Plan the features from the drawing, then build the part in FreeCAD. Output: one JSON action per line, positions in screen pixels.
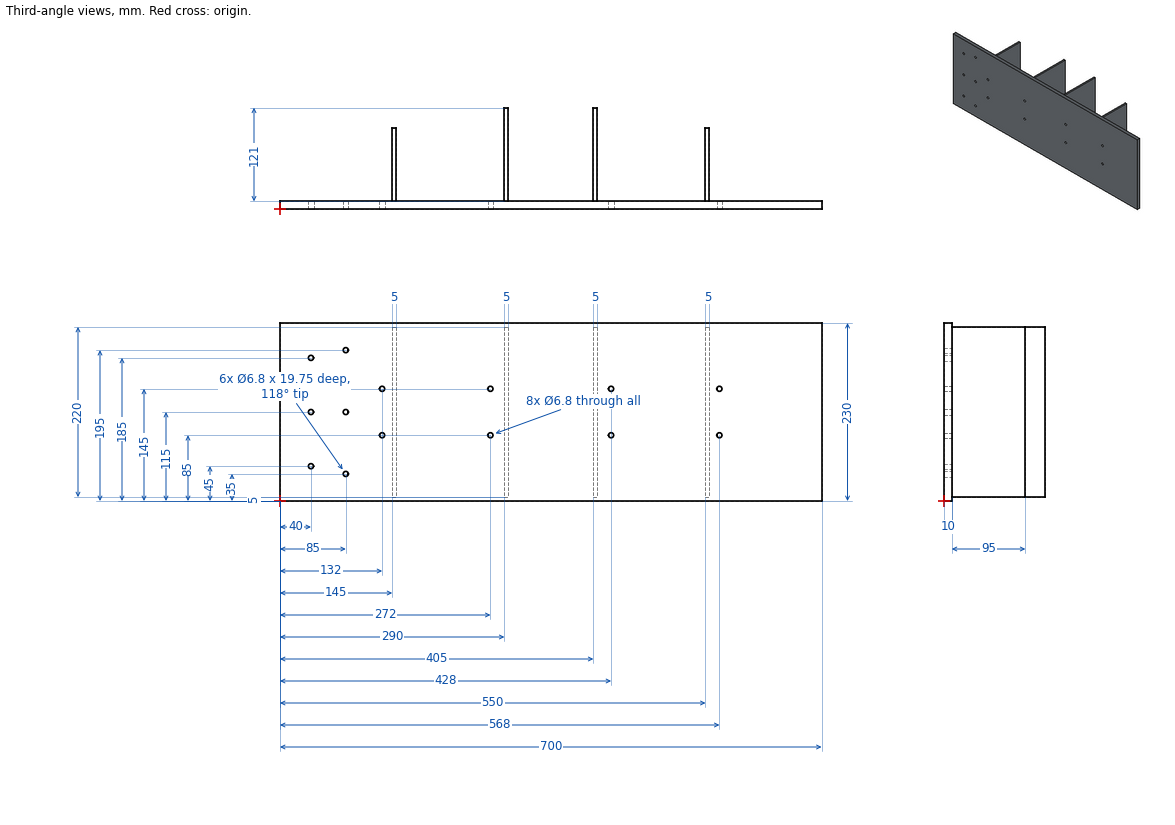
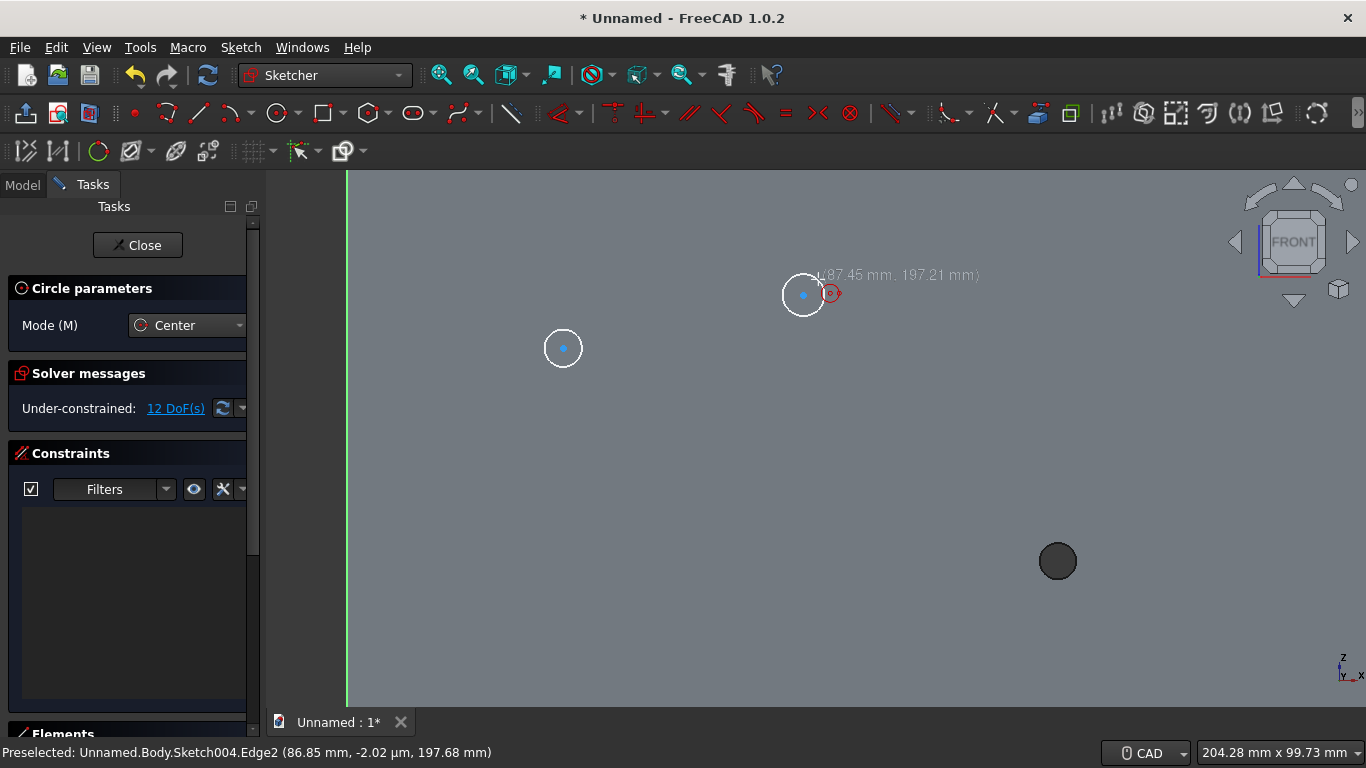
{"action": "scroll", "coordinate": [817, 279], "scroll_direction": "down", "scroll_amount": 6}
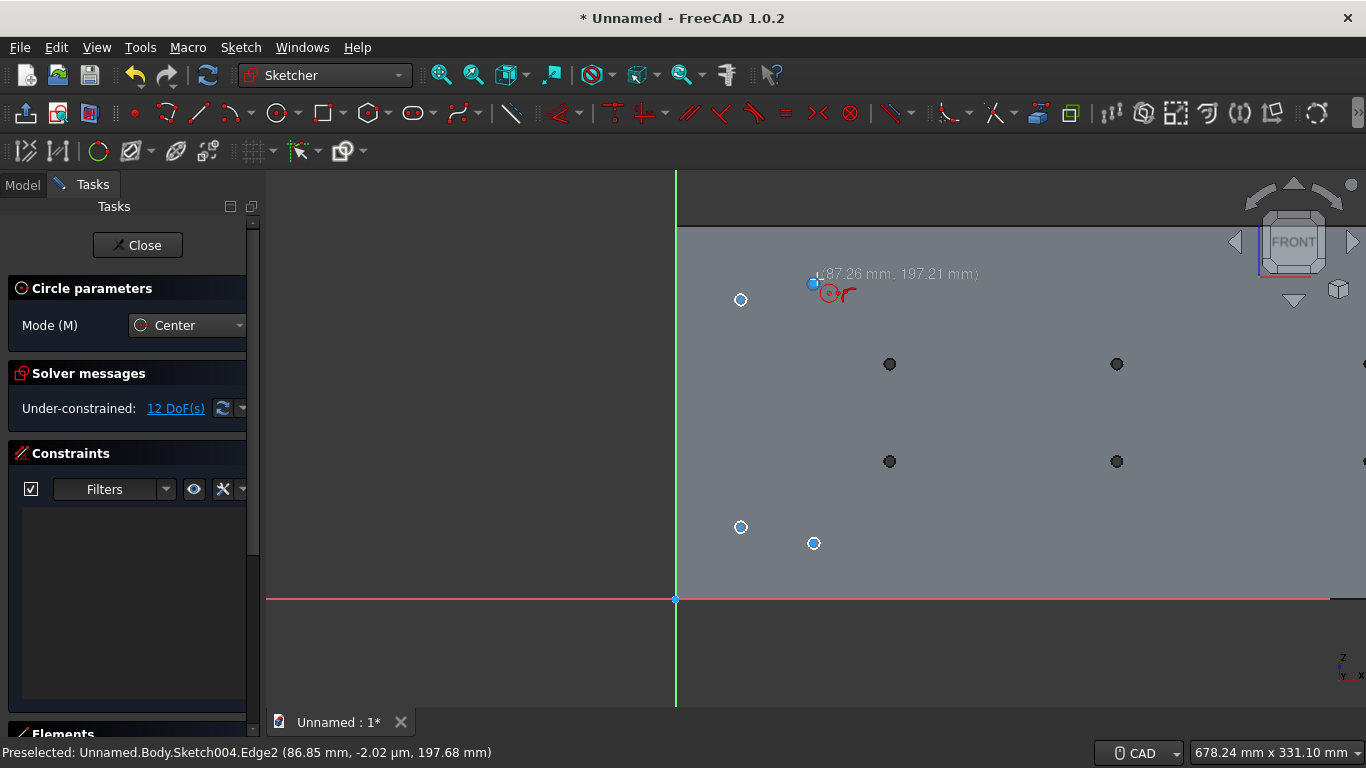
{"action": "scroll", "coordinate": [741, 413], "scroll_direction": "up", "scroll_amount": 8}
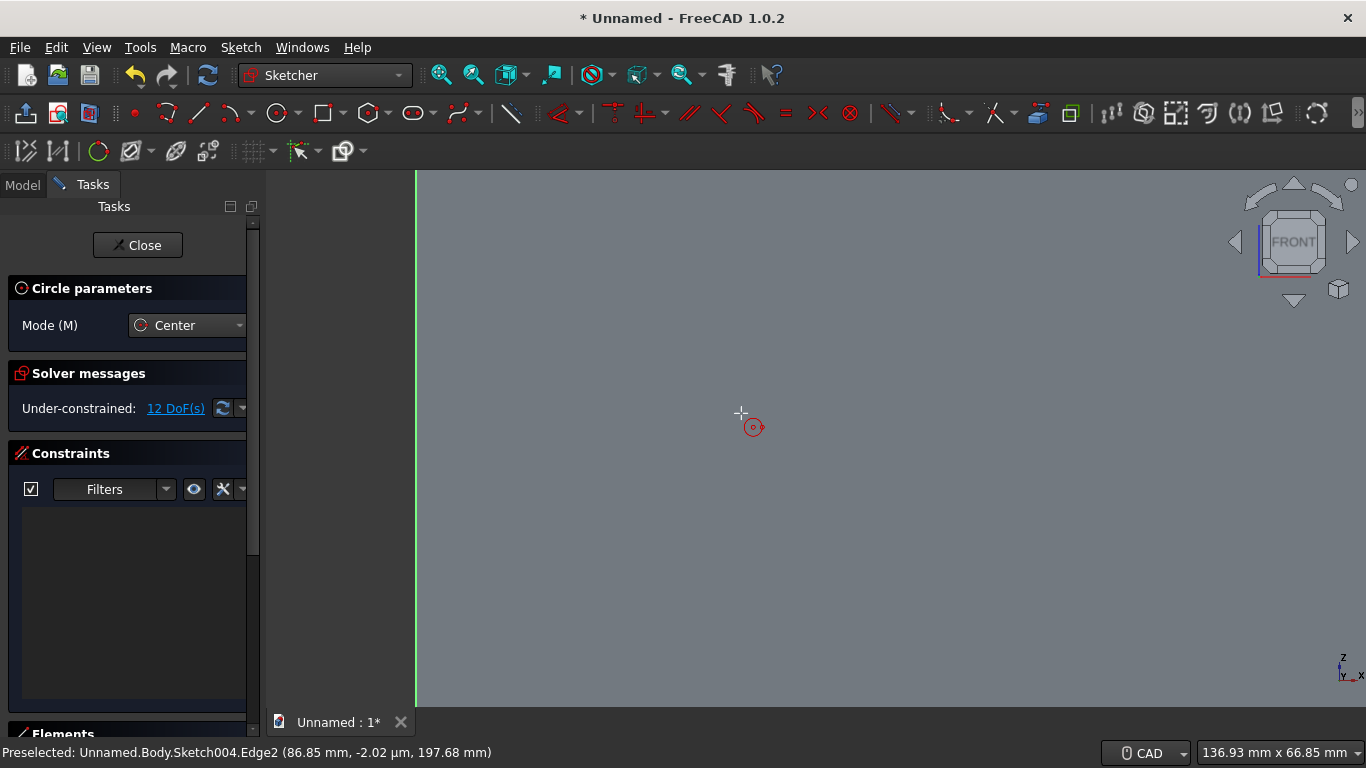
{"action": "scroll", "coordinate": [741, 414], "scroll_direction": "down", "scroll_amount": 8}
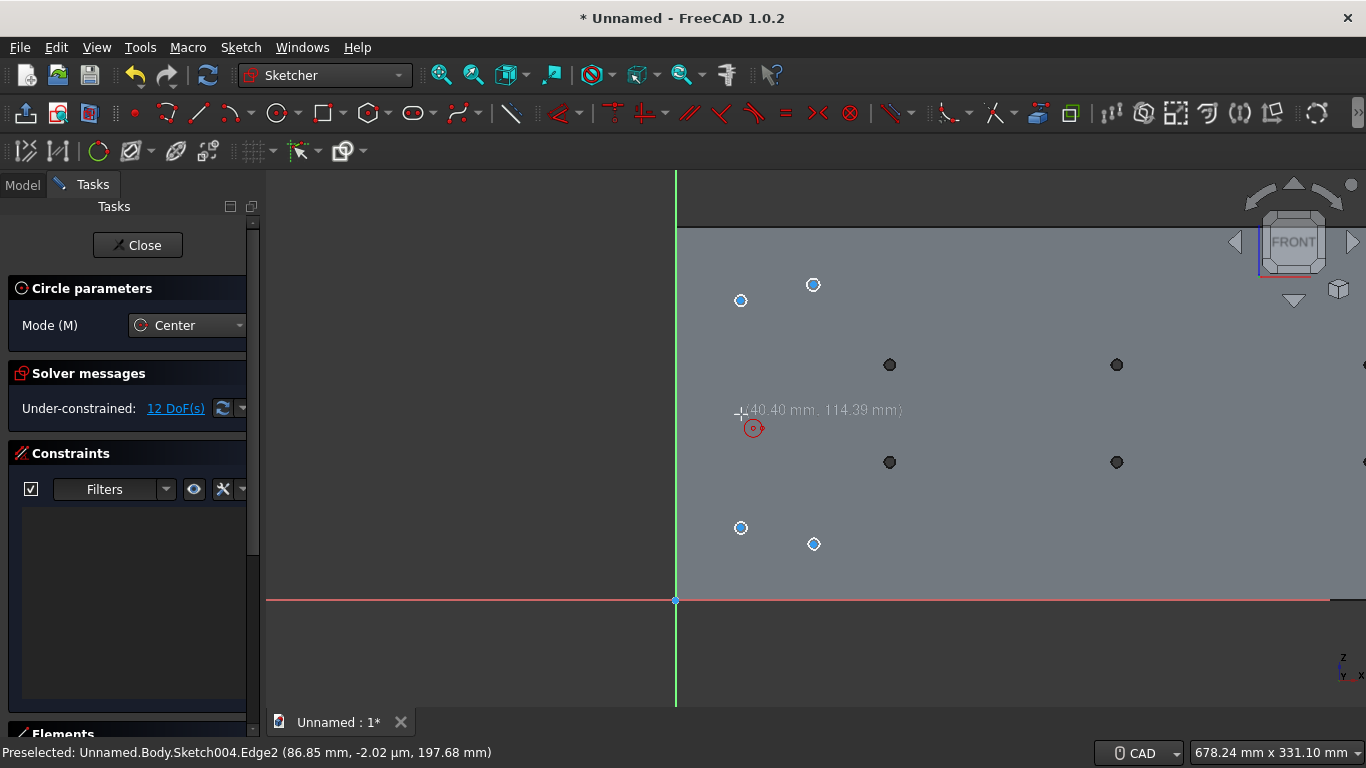
{"action": "left_click", "coordinate": [741, 414]}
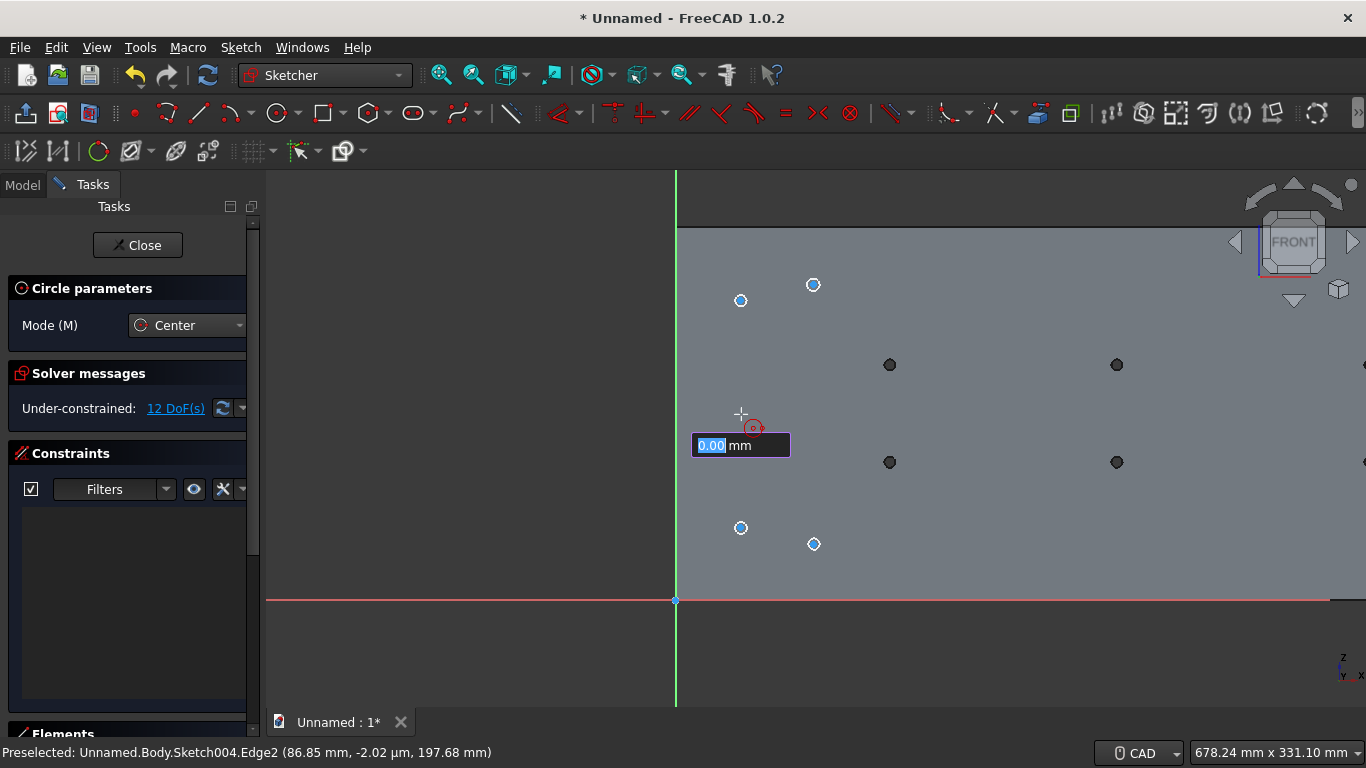
{"action": "scroll", "coordinate": [745, 410], "scroll_direction": "up", "scroll_amount": 6}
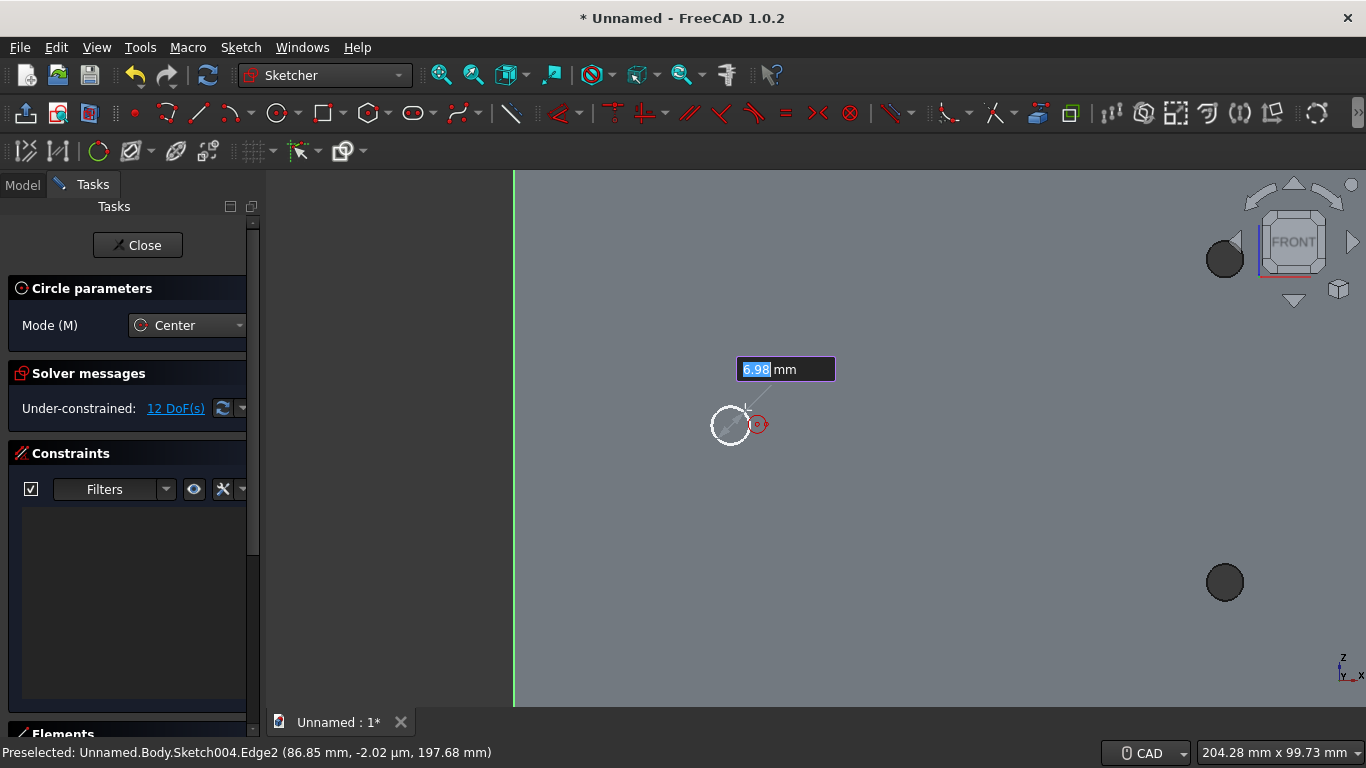
{"action": "left_click", "coordinate": [743, 408]}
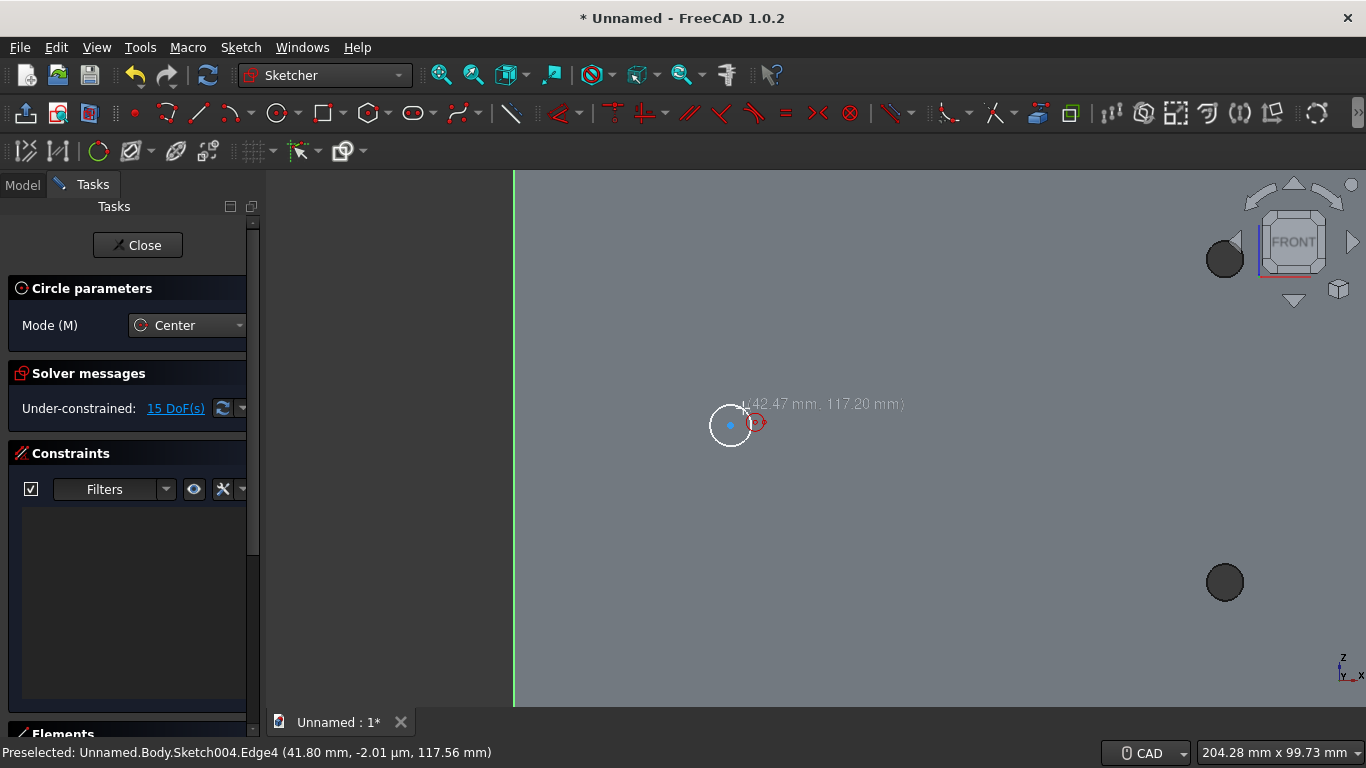
{"action": "scroll", "coordinate": [972, 421], "scroll_direction": "up", "scroll_amount": 2}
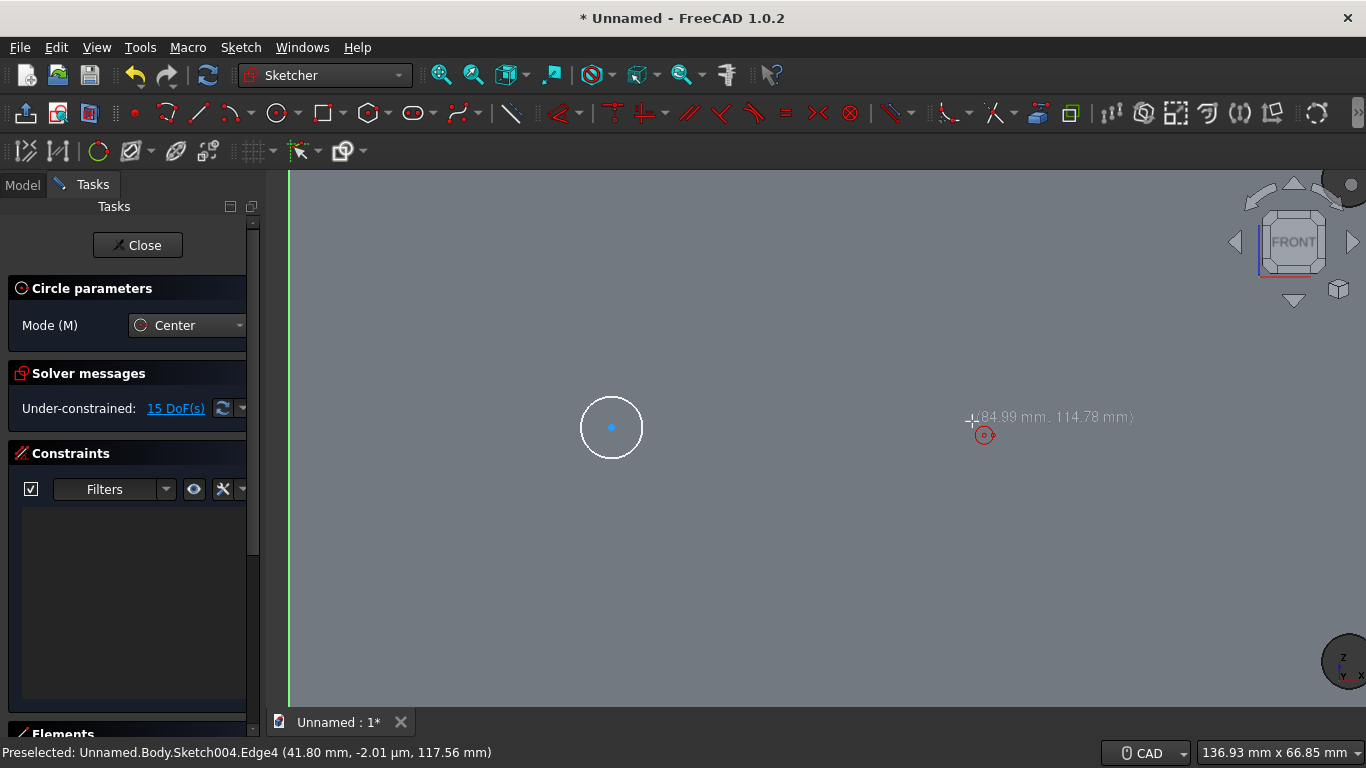
{"action": "scroll", "coordinate": [774, 411], "scroll_direction": "down", "scroll_amount": 8}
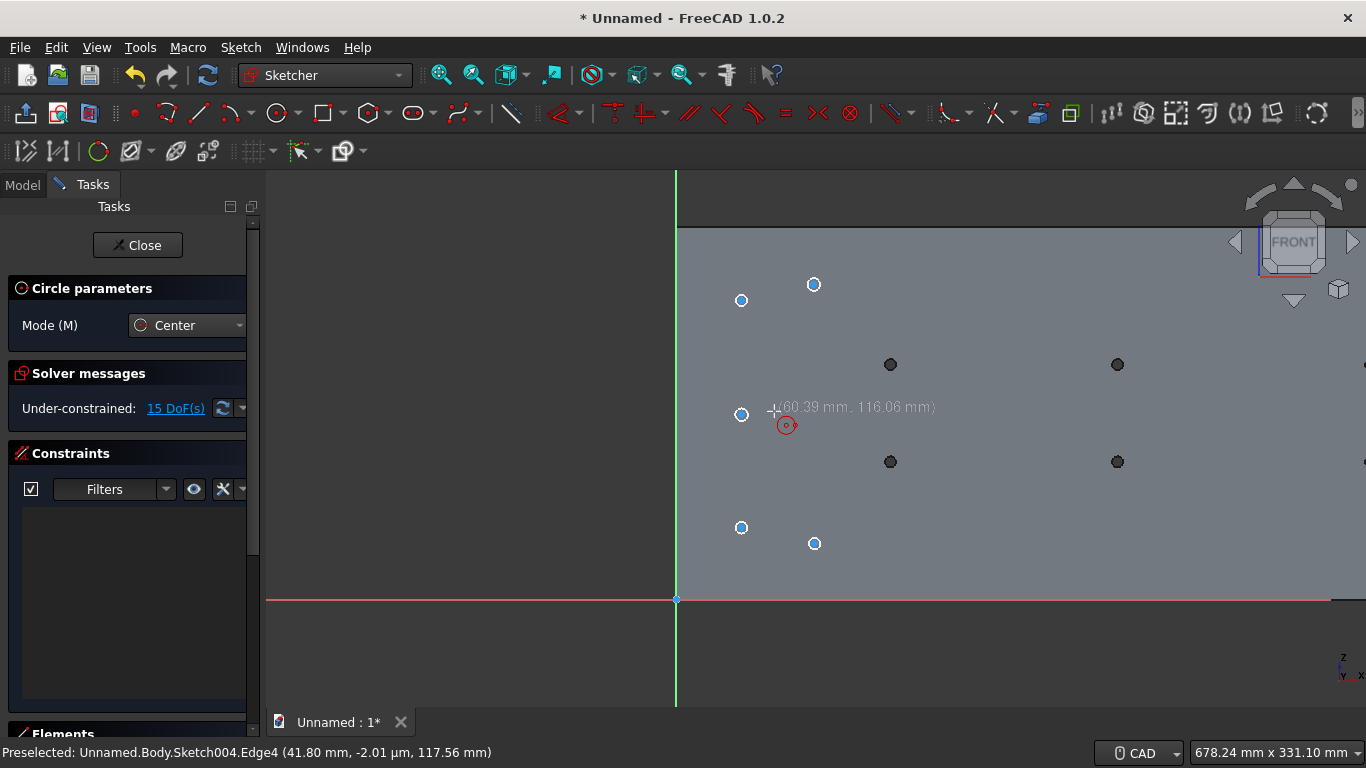
{"action": "left_click", "coordinate": [814, 413]}